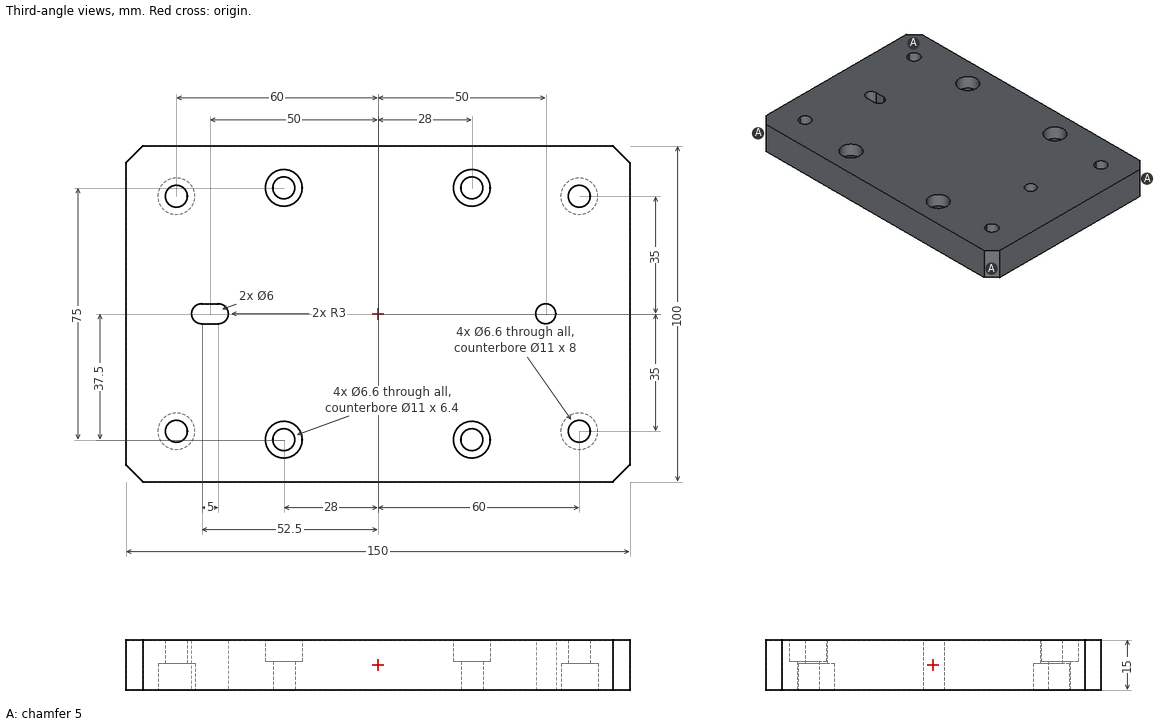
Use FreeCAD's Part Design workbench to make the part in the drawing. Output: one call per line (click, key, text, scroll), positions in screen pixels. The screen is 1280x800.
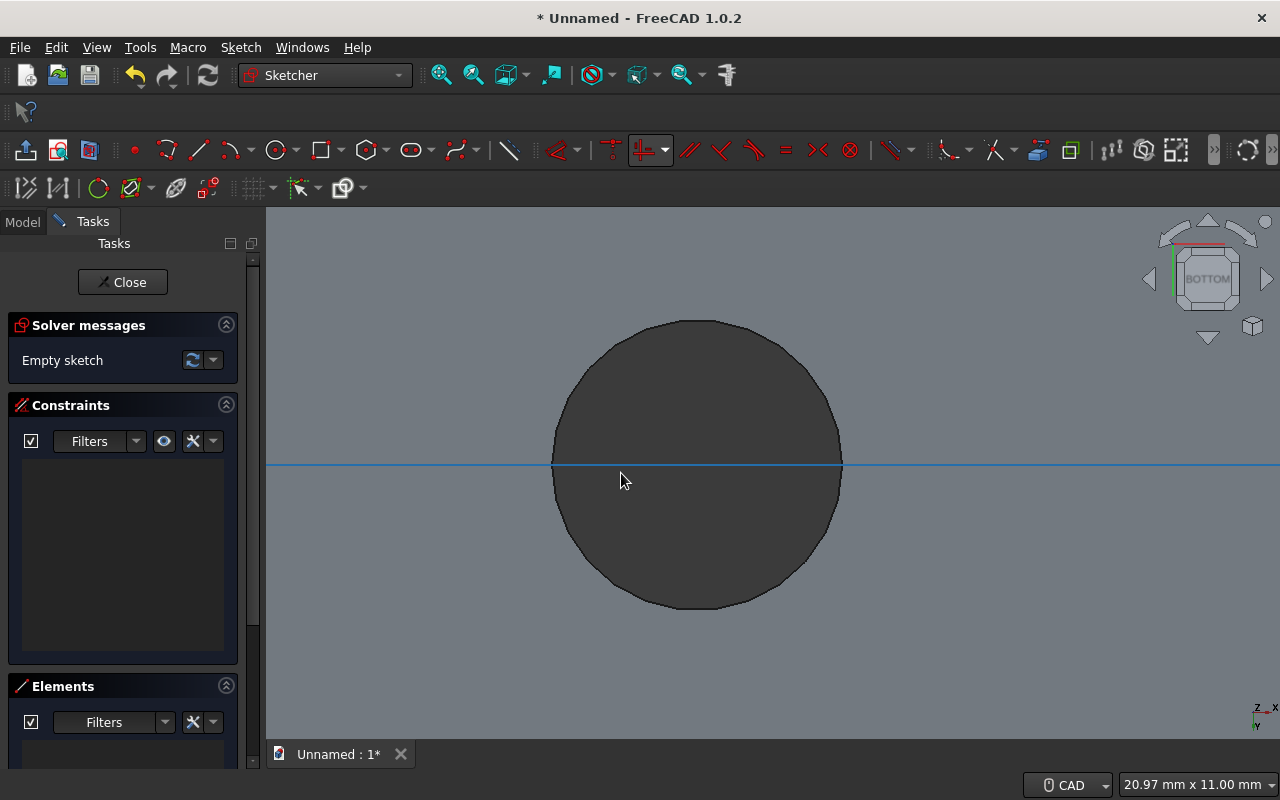
key(g)
key(s)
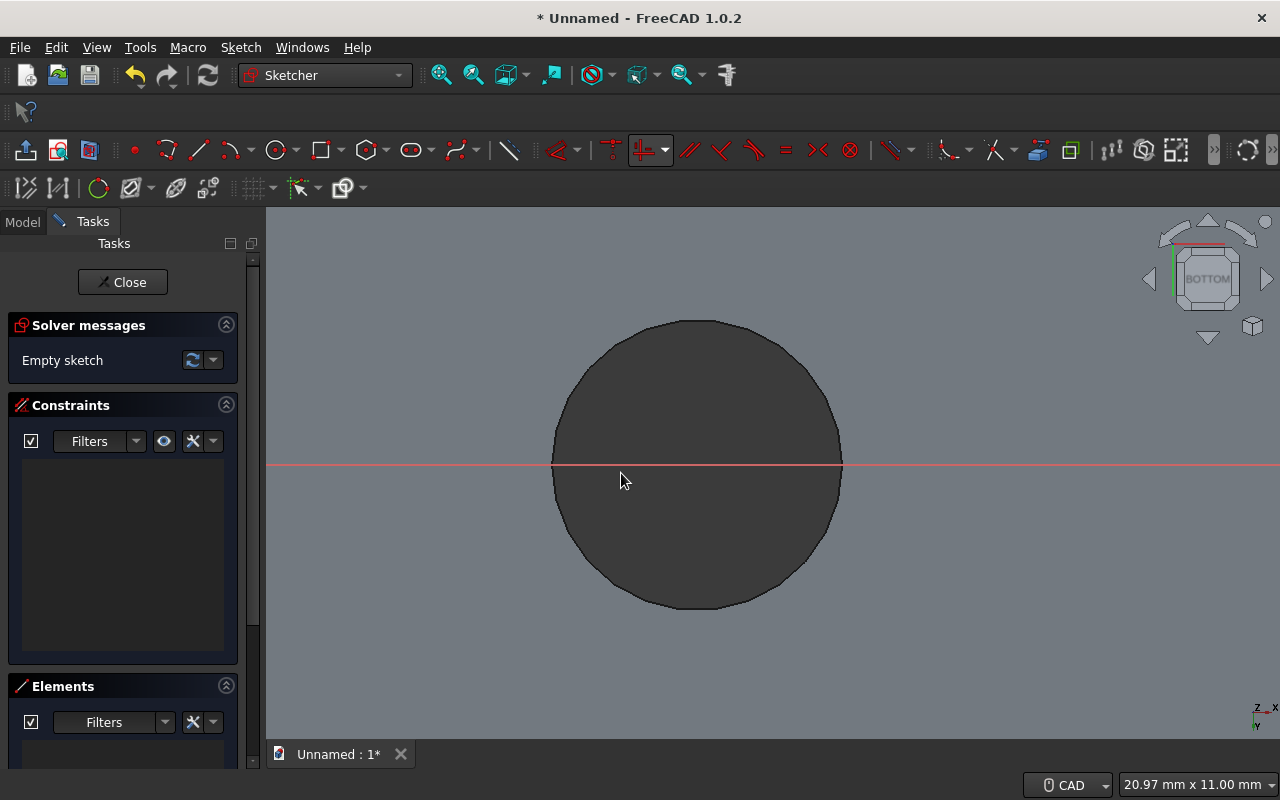
click(576, 465)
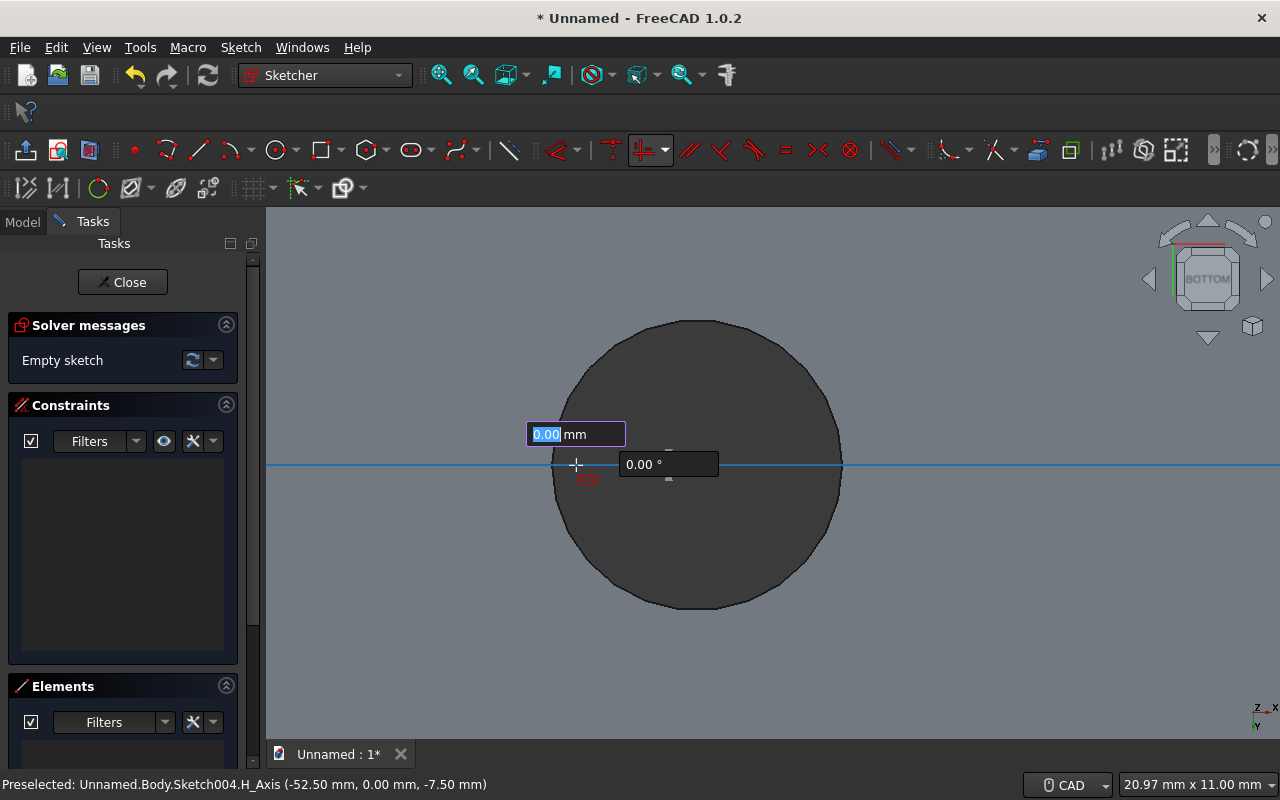
click(818, 456)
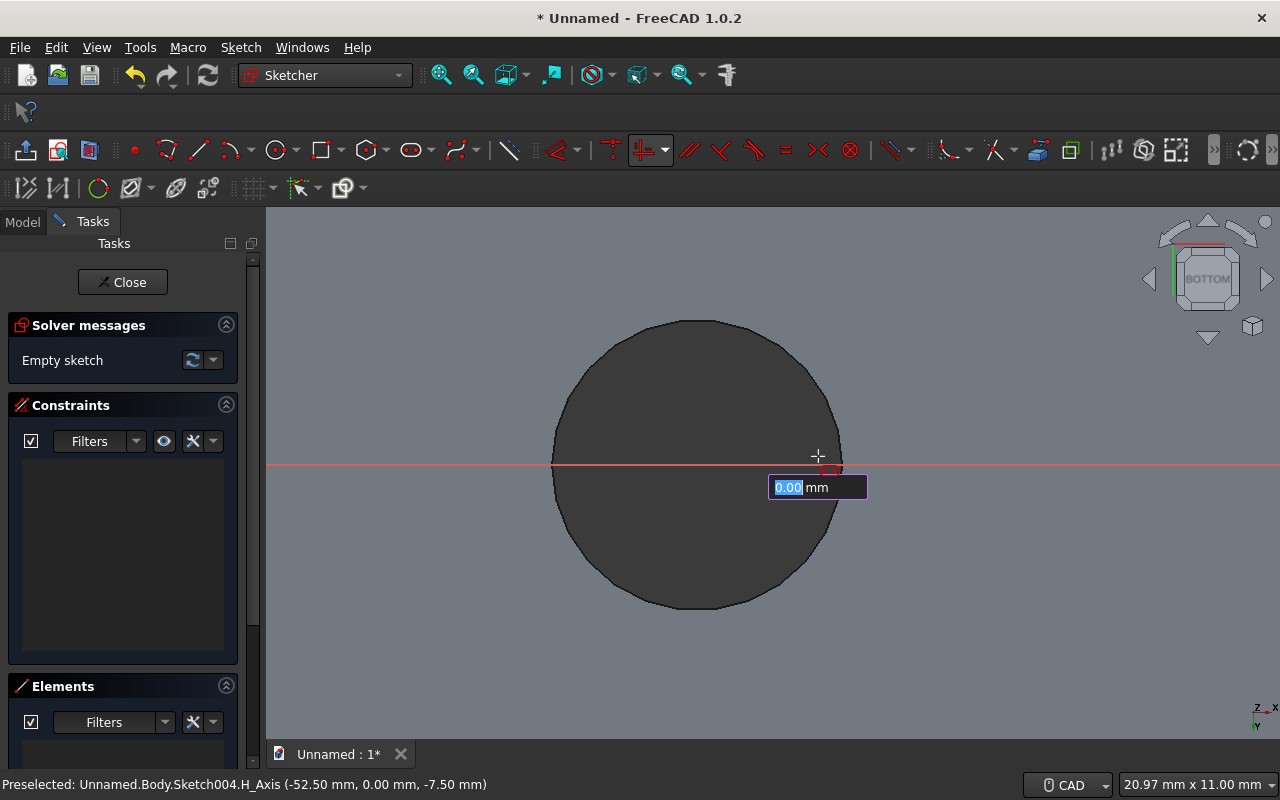
click(697, 610)
key(Escape)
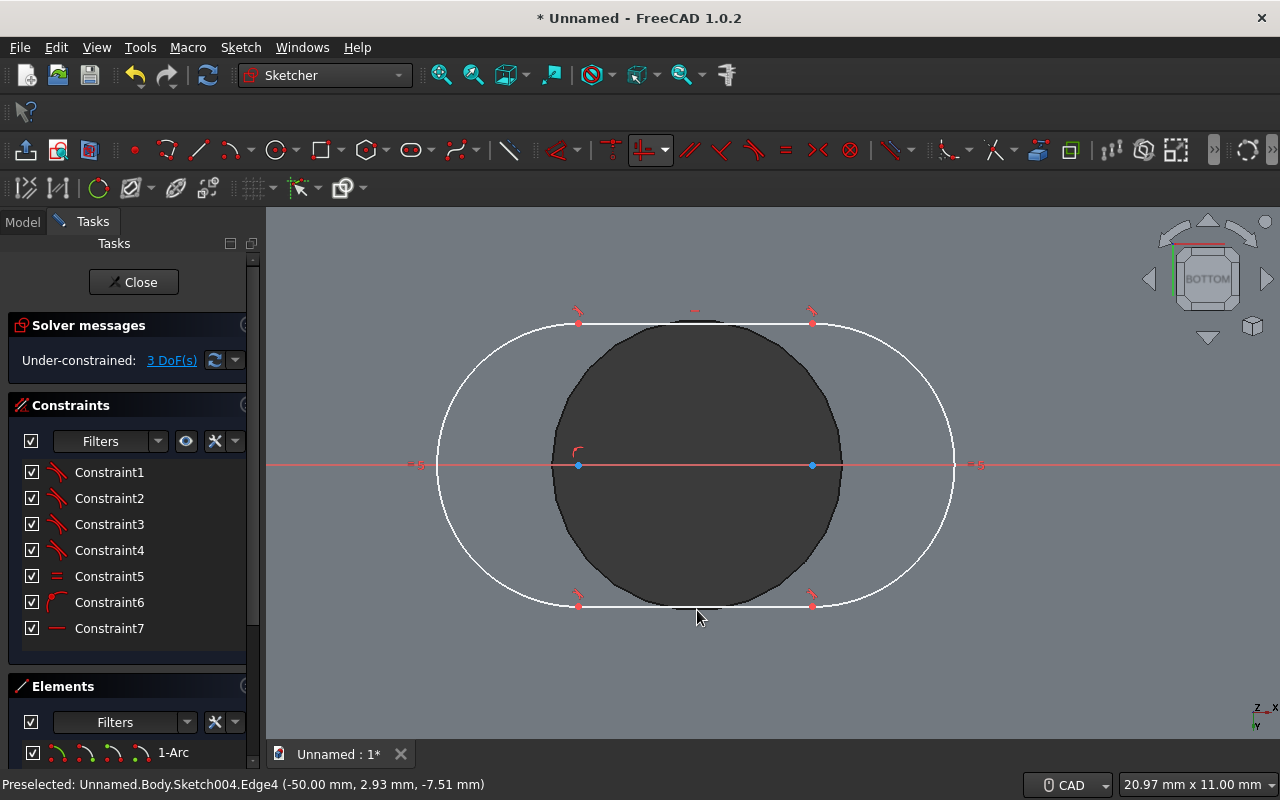
click(556, 150)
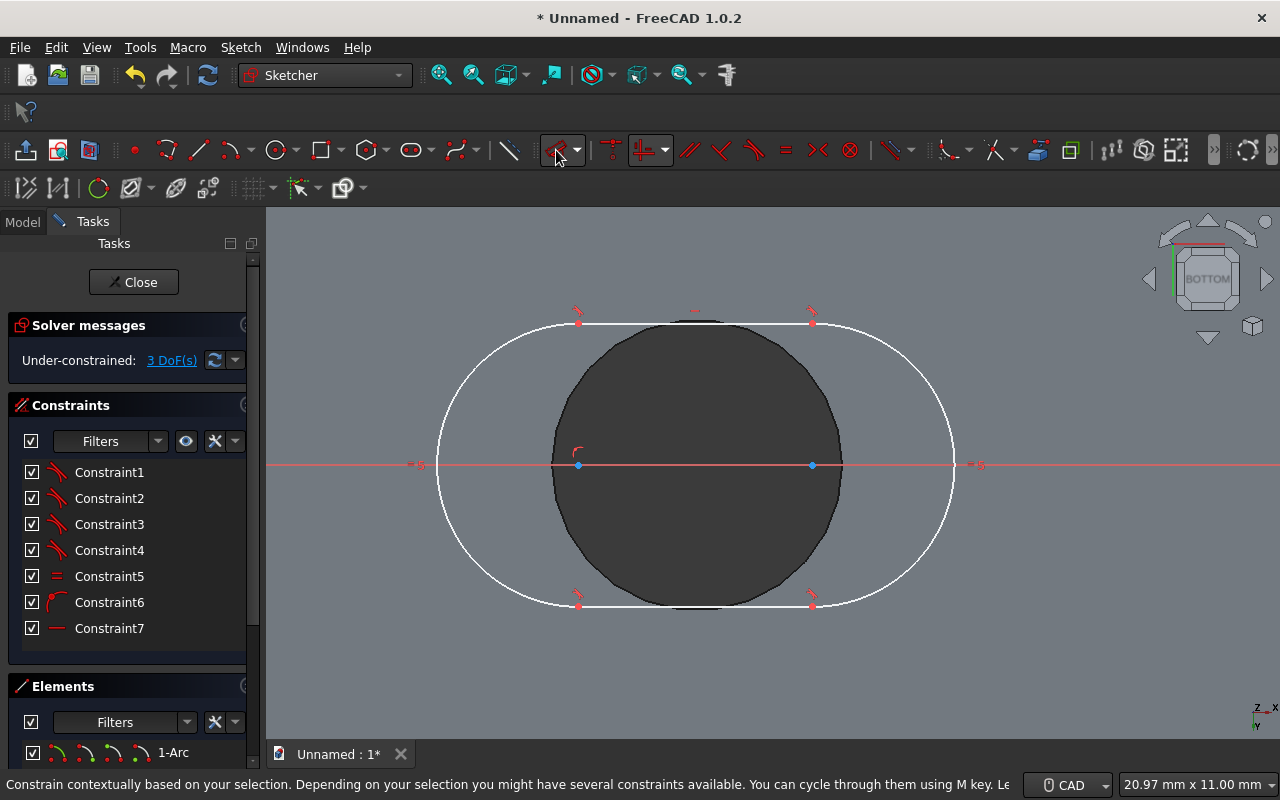
click(464, 382)
click(438, 363)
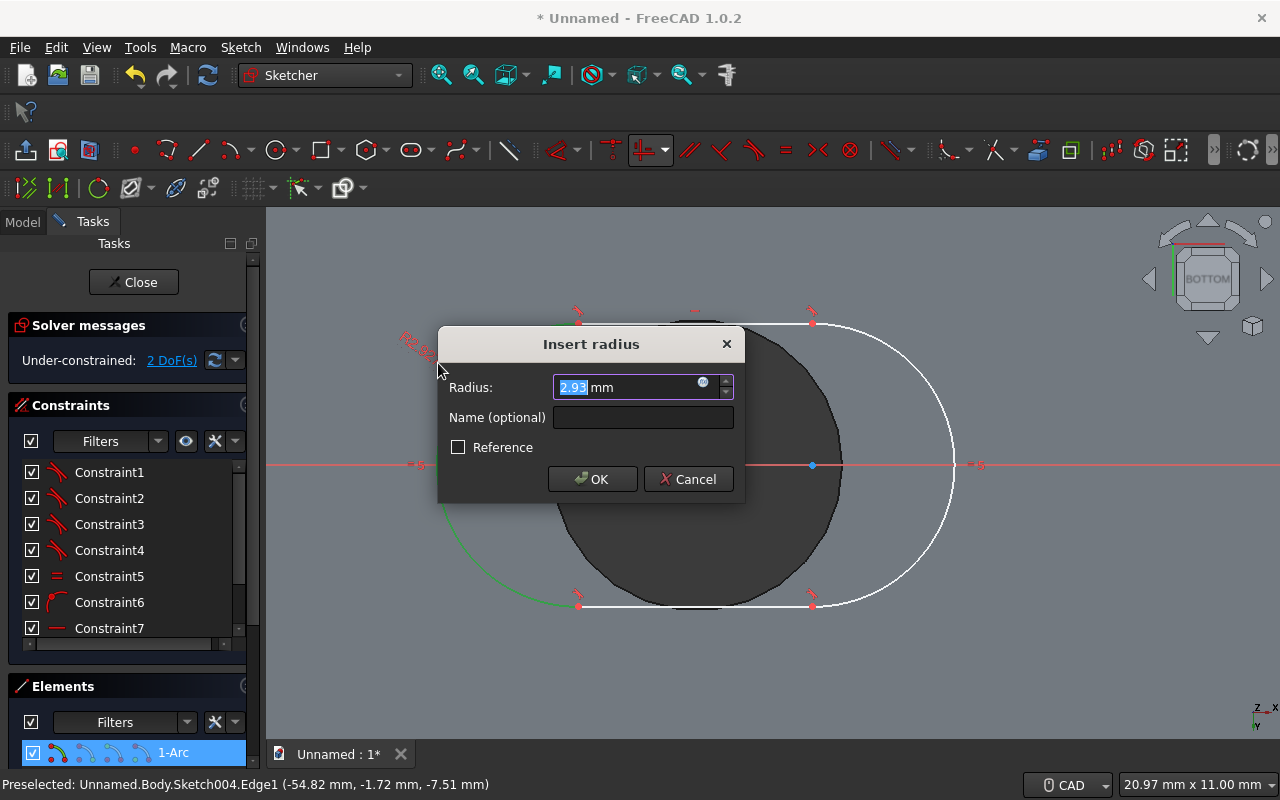
text(3)
key(Return)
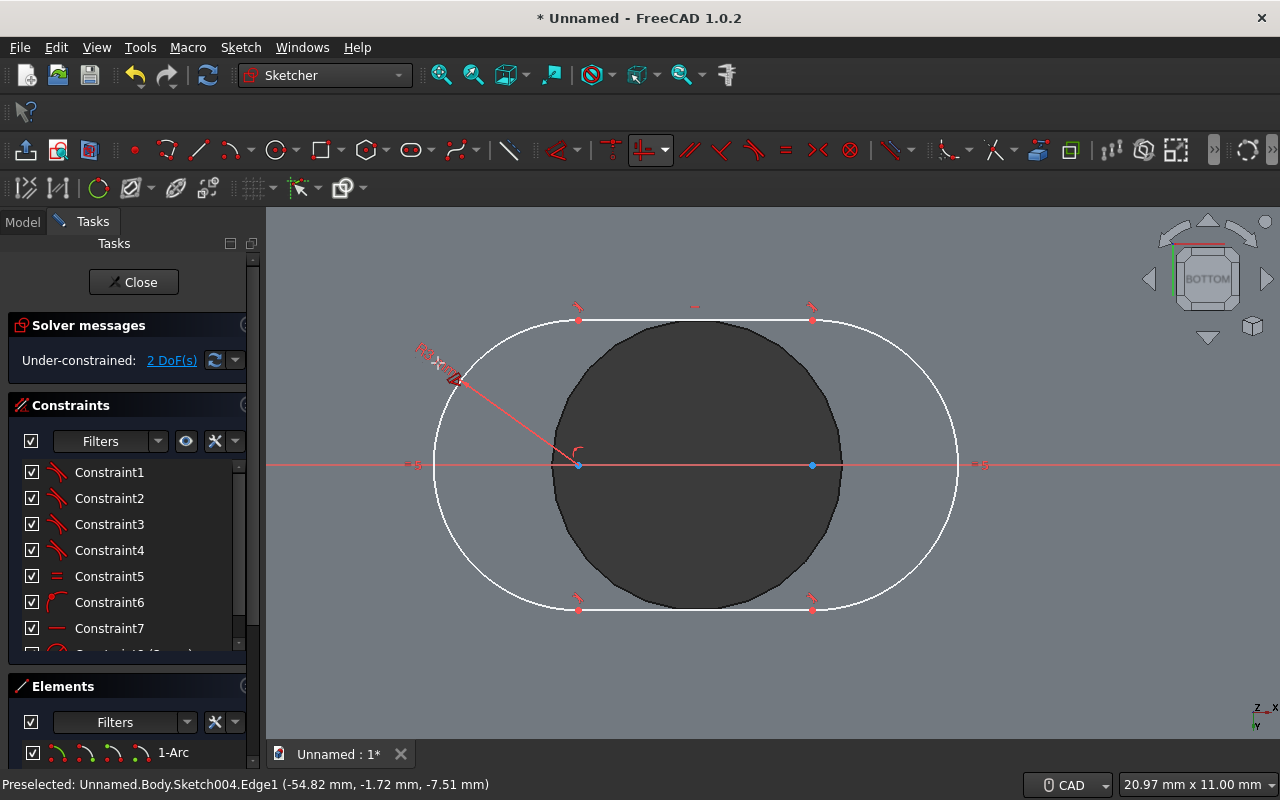
click(649, 320)
click(696, 286)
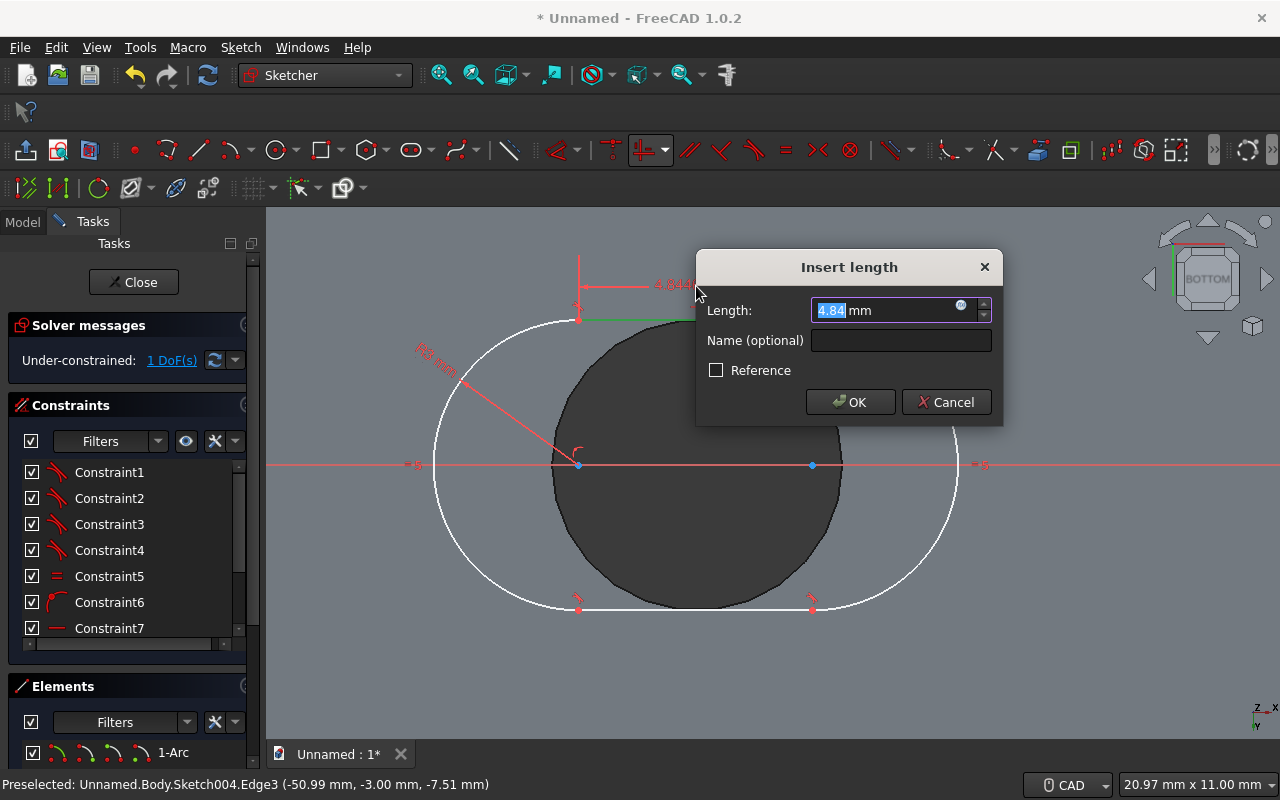
text(5)
key(Return)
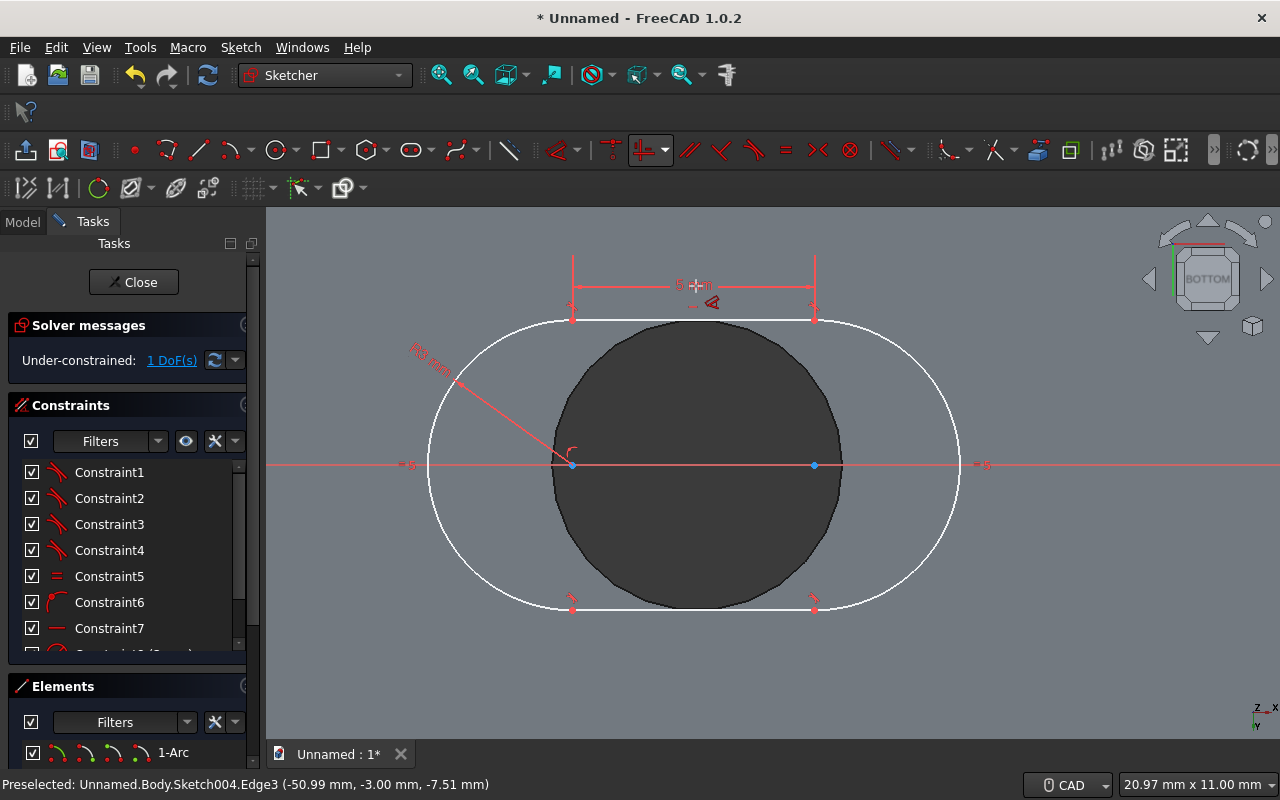
click(573, 320)
click(844, 286)